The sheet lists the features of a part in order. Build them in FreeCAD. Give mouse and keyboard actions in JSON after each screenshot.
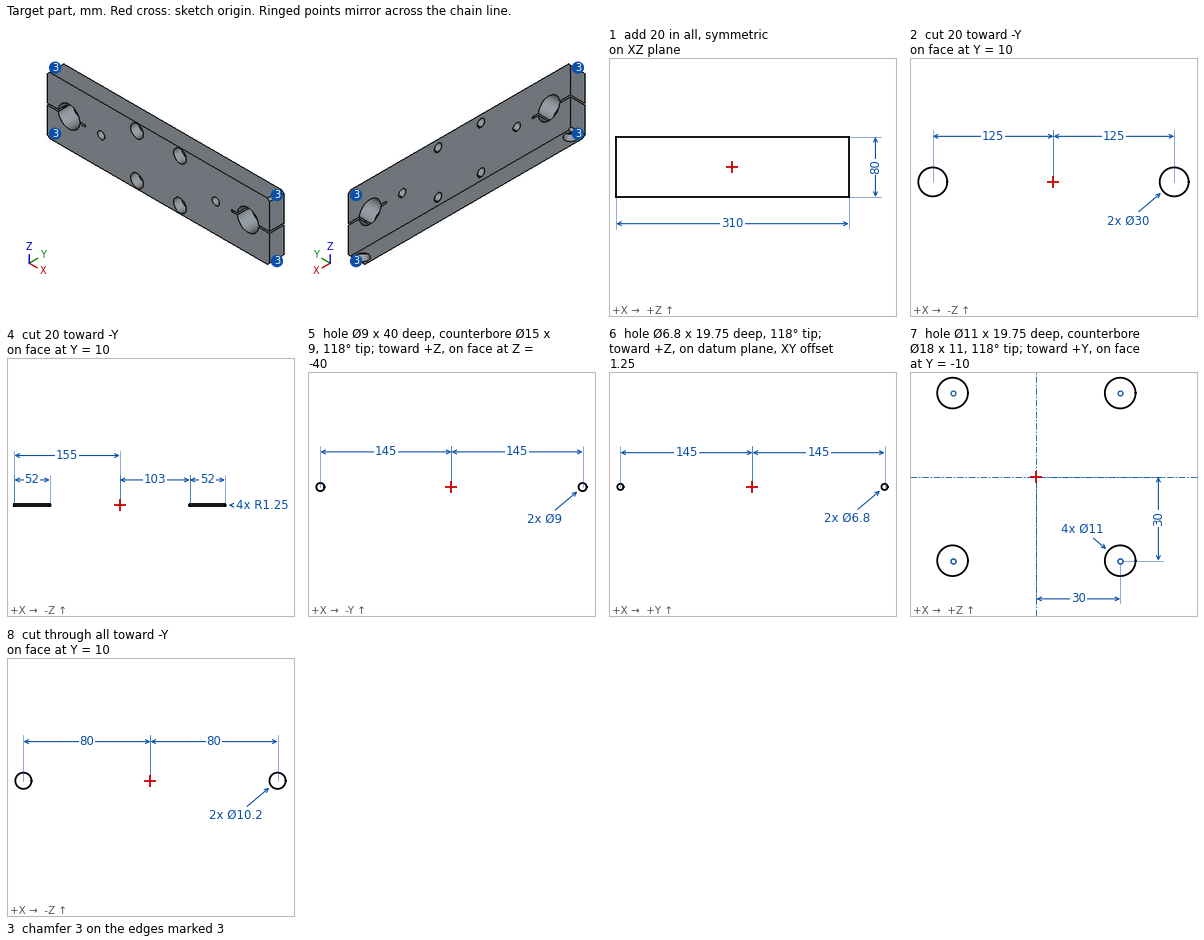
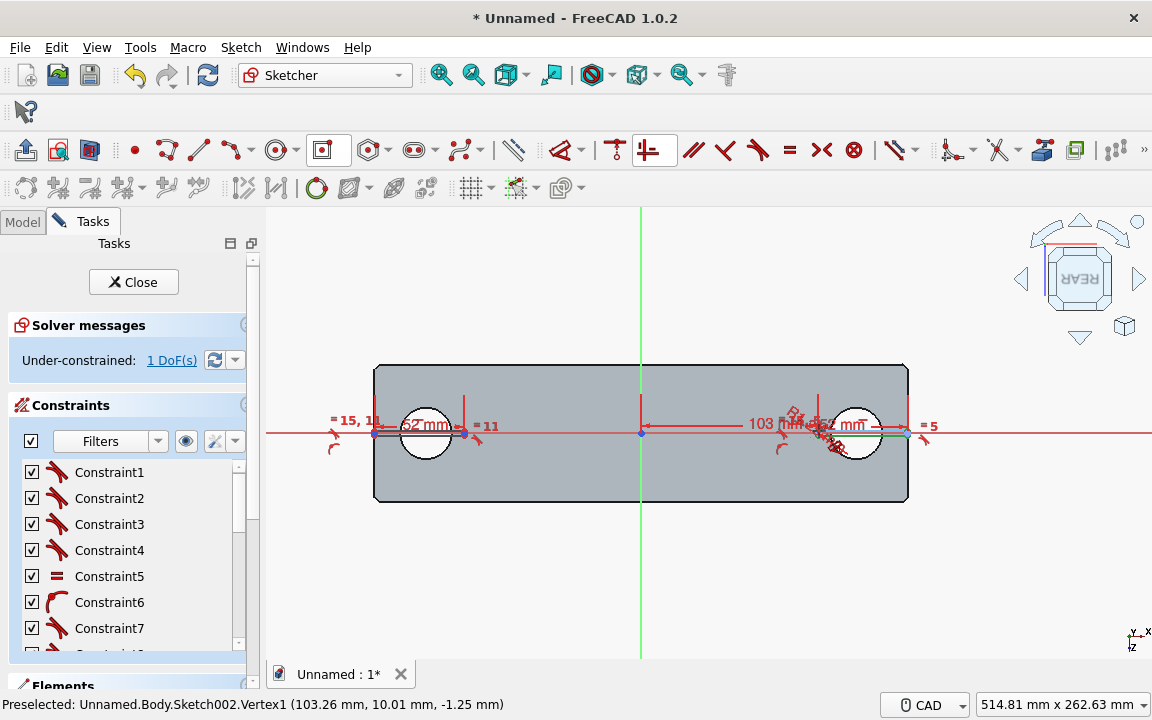
{"action": "scroll", "coordinate": [375, 431], "scroll_direction": "up", "scroll_amount": 9}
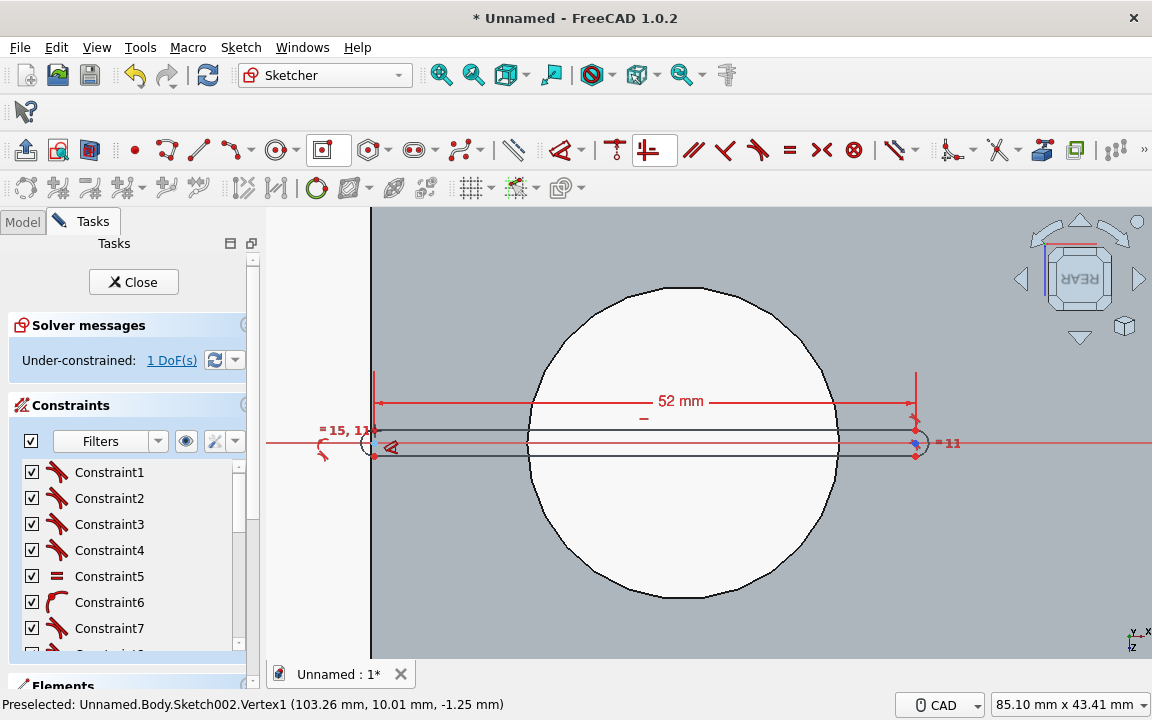
{"action": "left_click", "coordinate": [374, 430]}
{"action": "left_click", "coordinate": [540, 396]}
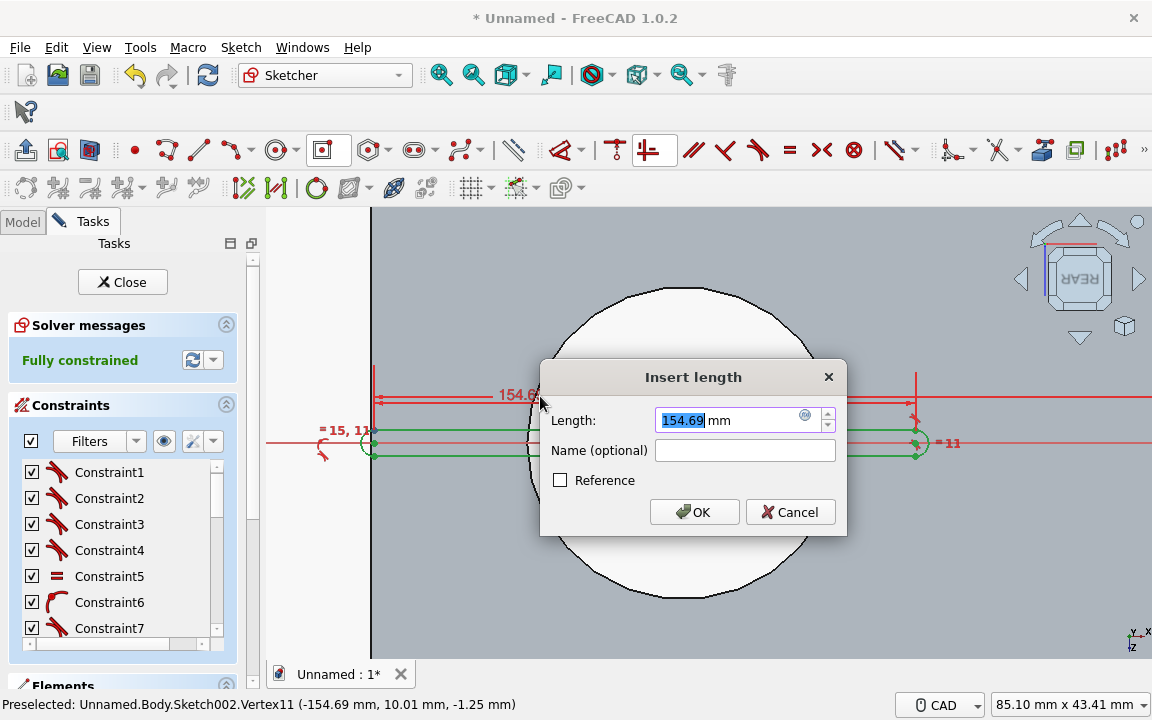
{"action": "type", "text": "155"}
{"action": "key", "text": "Return"}
{"action": "key", "text": "Escape"}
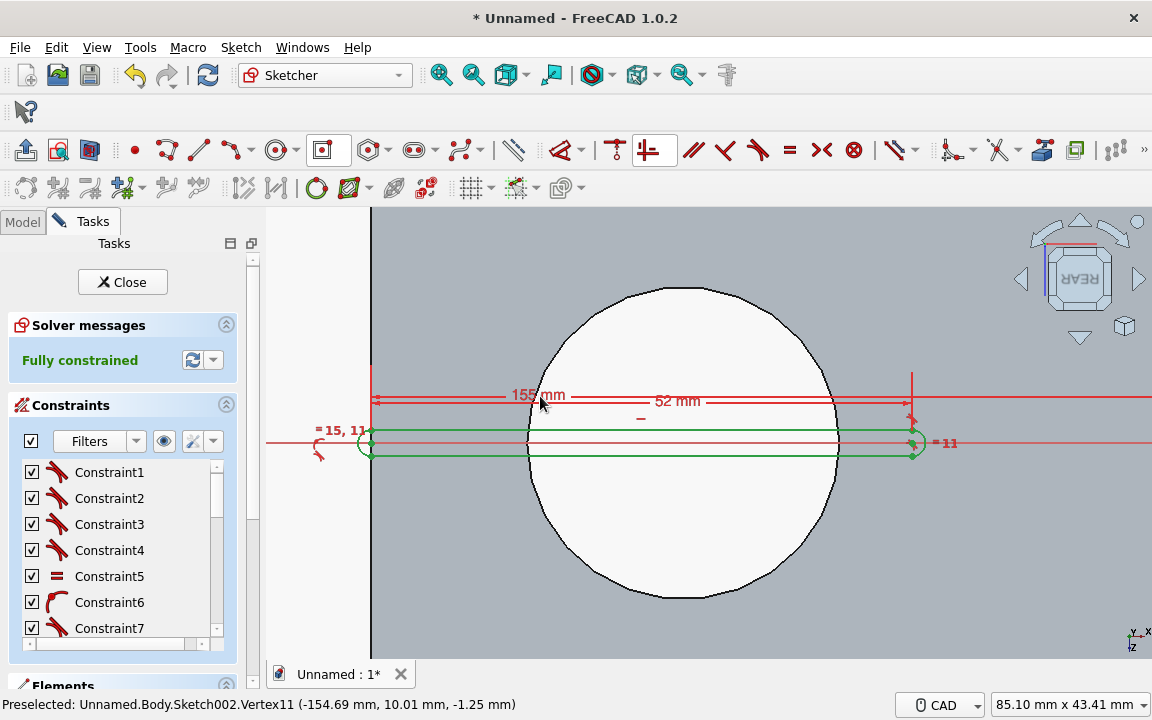
{"action": "left_click", "coordinate": [123, 282]}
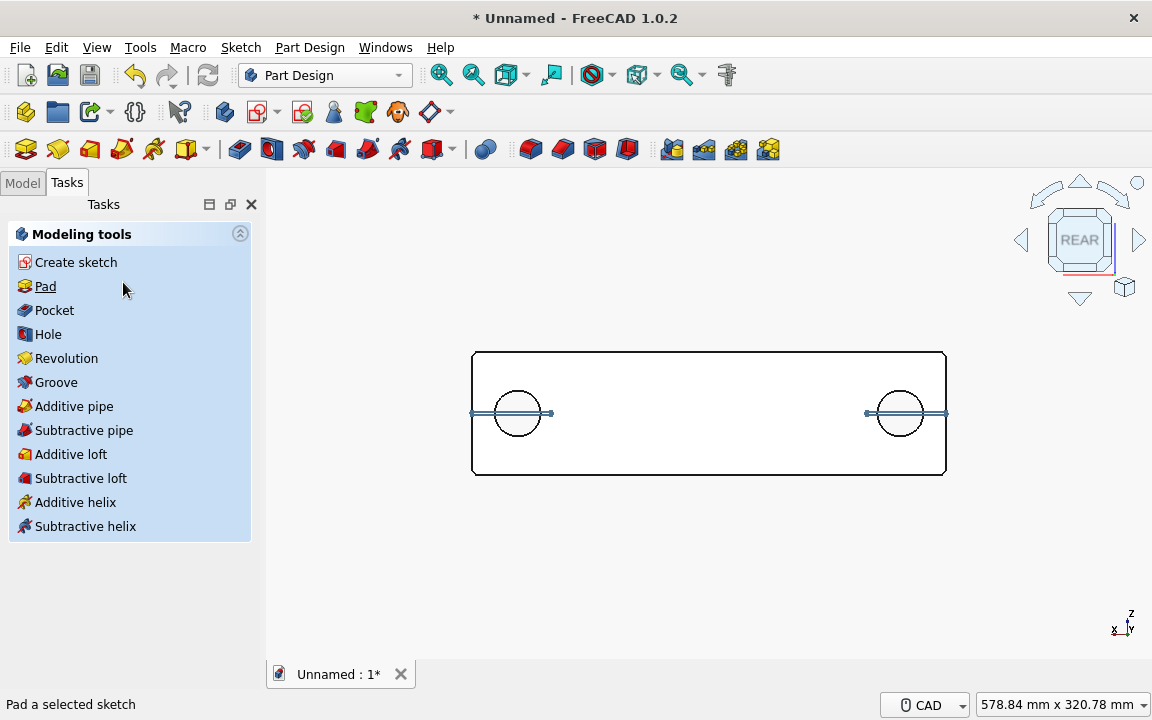
{"action": "left_click", "coordinate": [240, 150]}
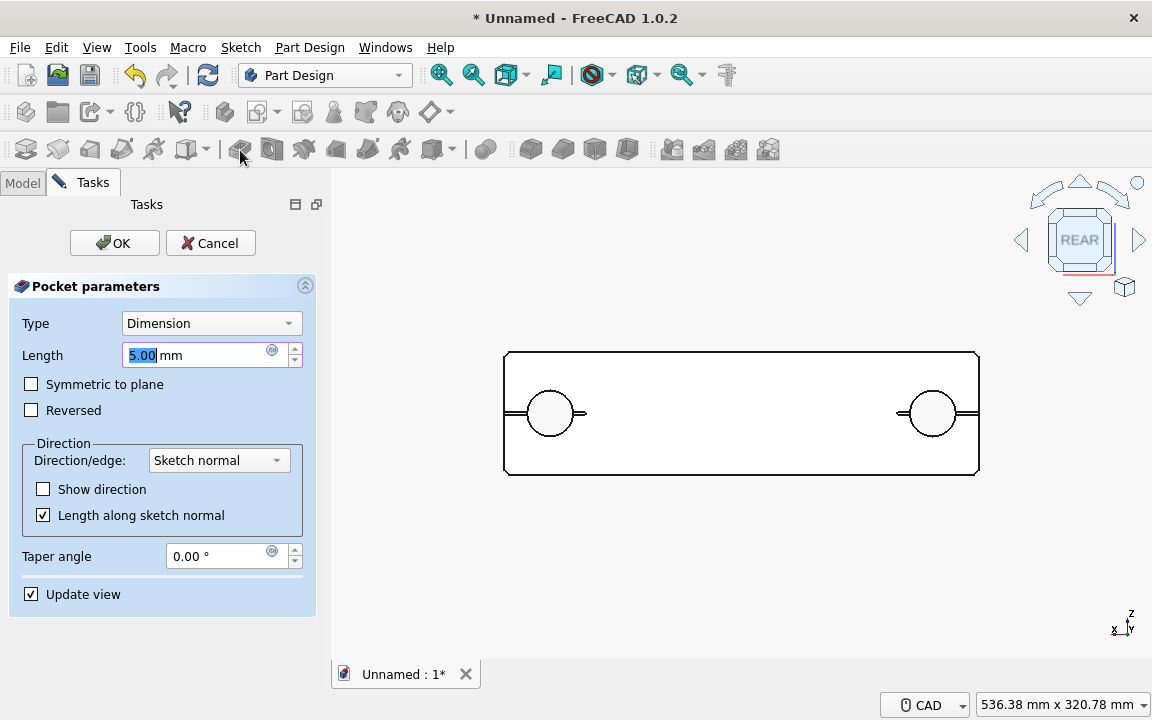
{"action": "type", "text": "20"}
{"action": "key", "text": "Tab"}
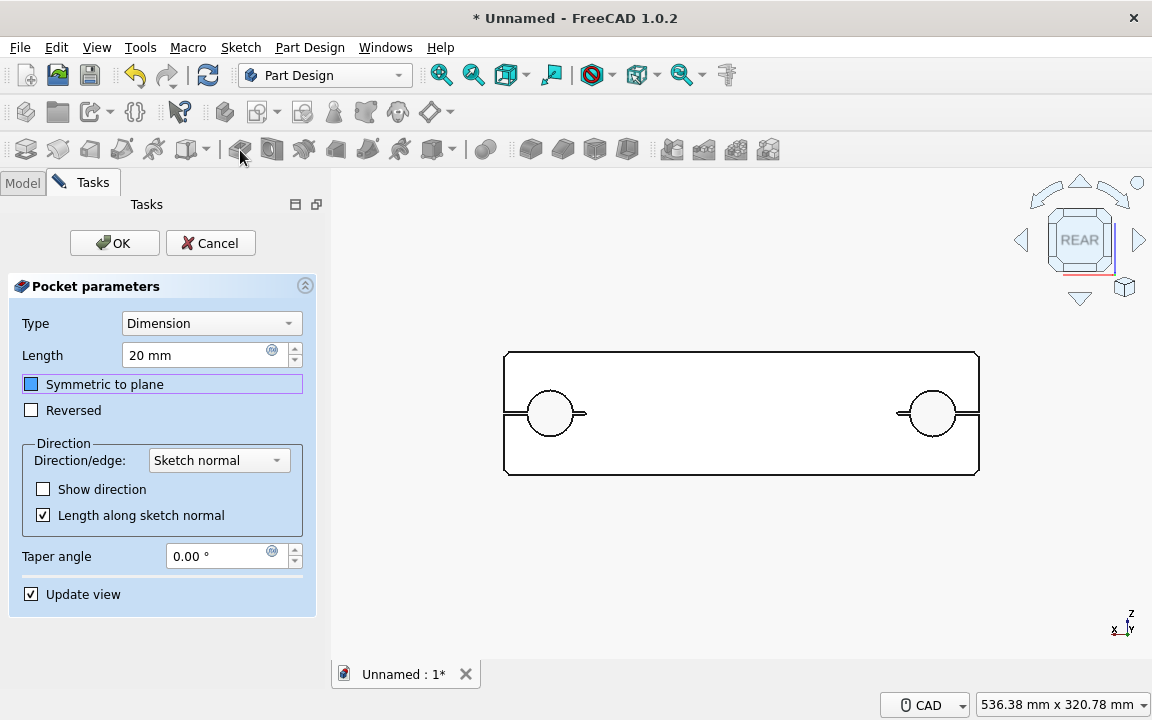
{"action": "left_click", "coordinate": [115, 243]}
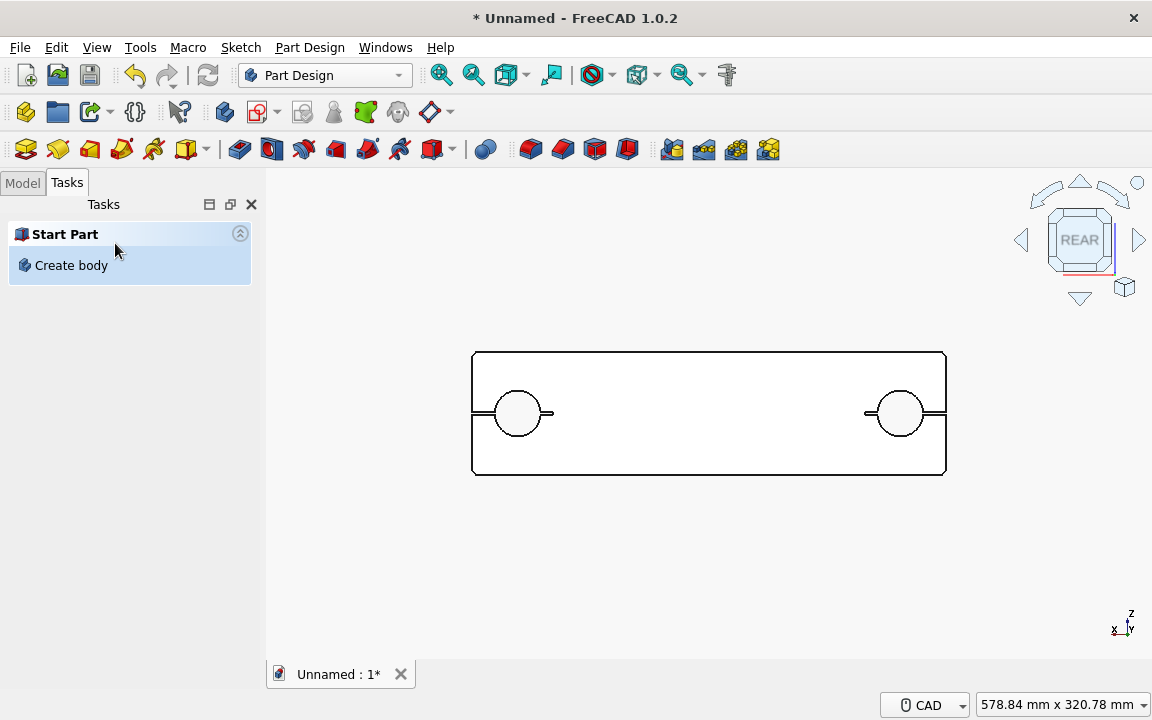
{"action": "key", "text": "5"}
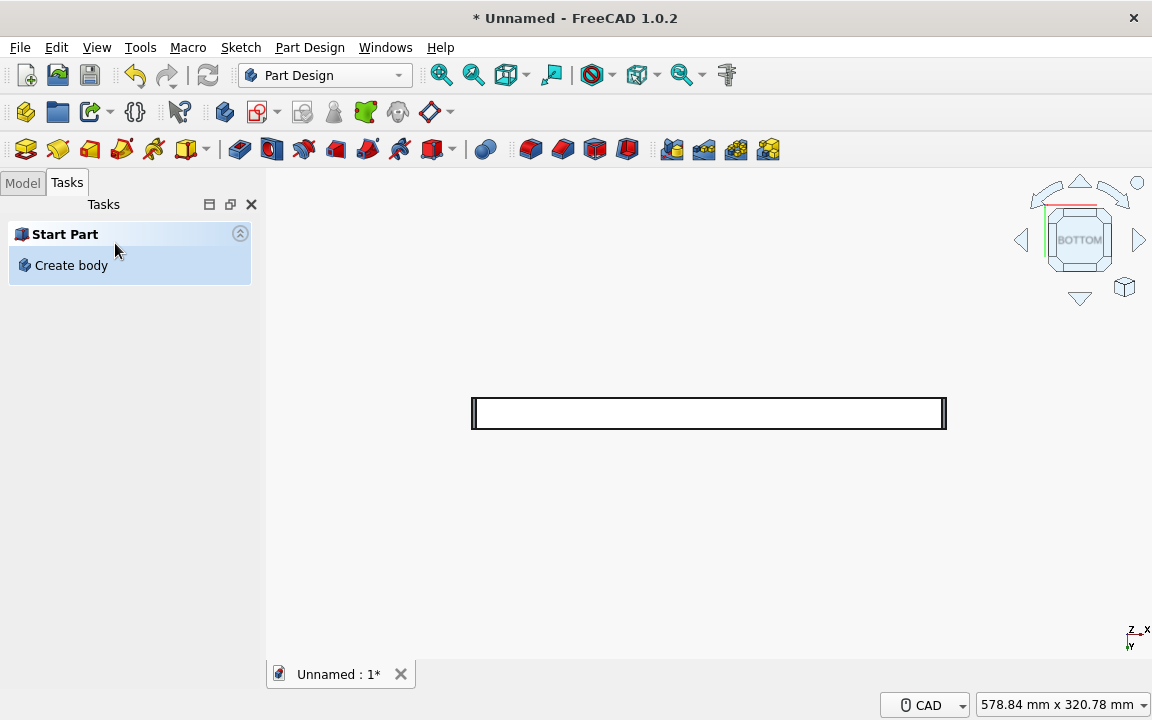
{"action": "left_click", "coordinate": [908, 413]}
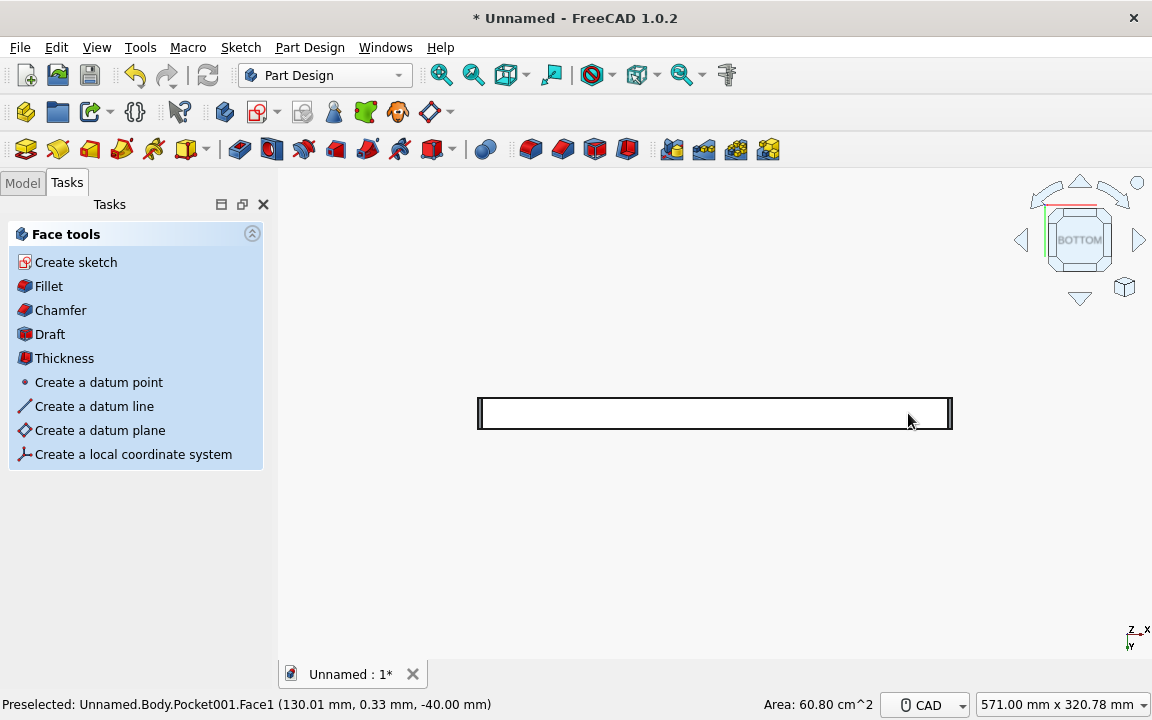
{"action": "left_click", "coordinate": [258, 112]}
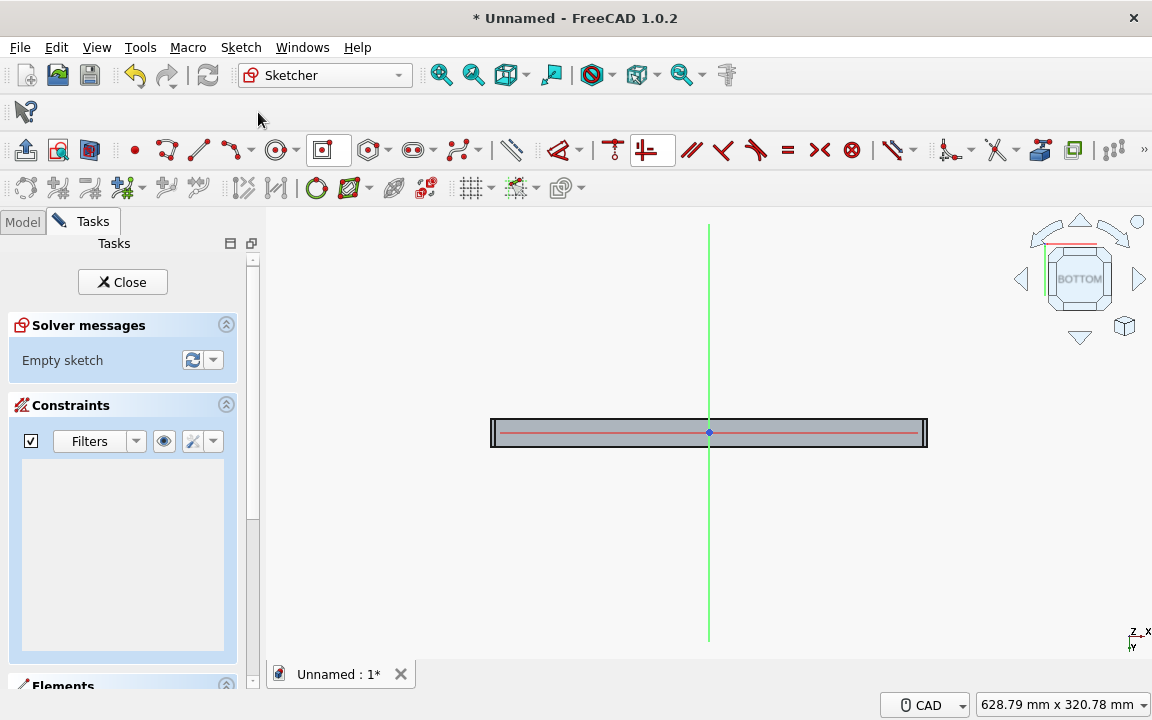
{"action": "left_click", "coordinate": [276, 150]}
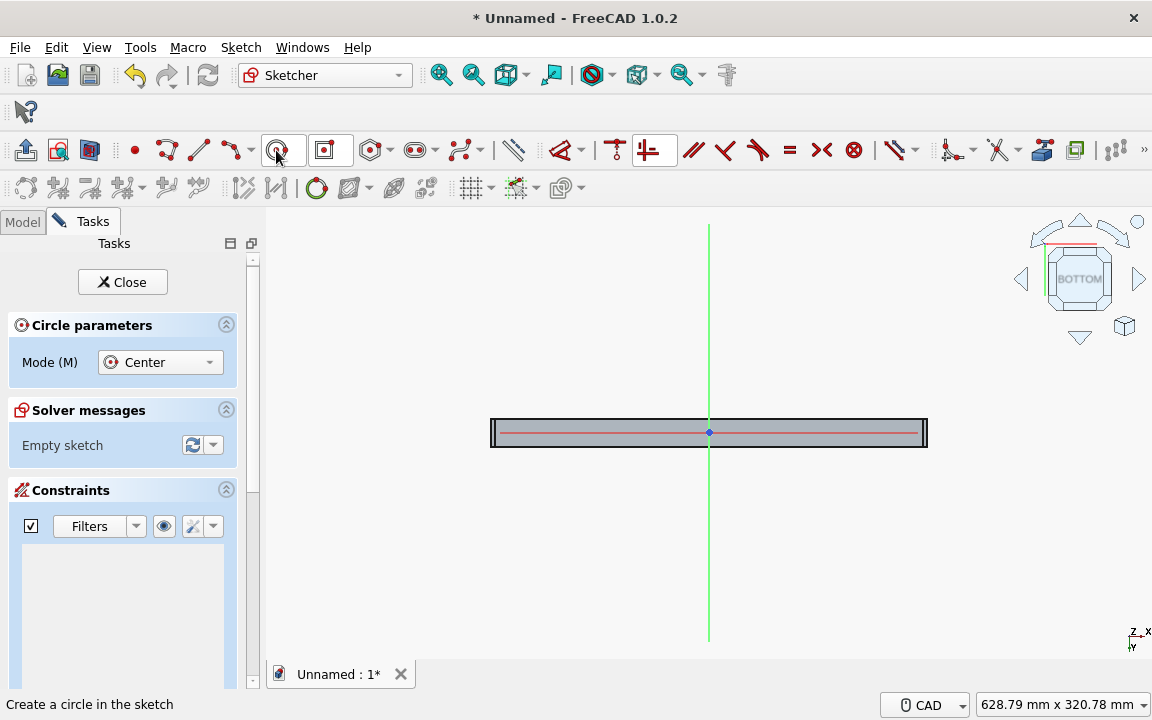
{"action": "scroll", "coordinate": [913, 433], "scroll_direction": "up", "scroll_amount": 7}